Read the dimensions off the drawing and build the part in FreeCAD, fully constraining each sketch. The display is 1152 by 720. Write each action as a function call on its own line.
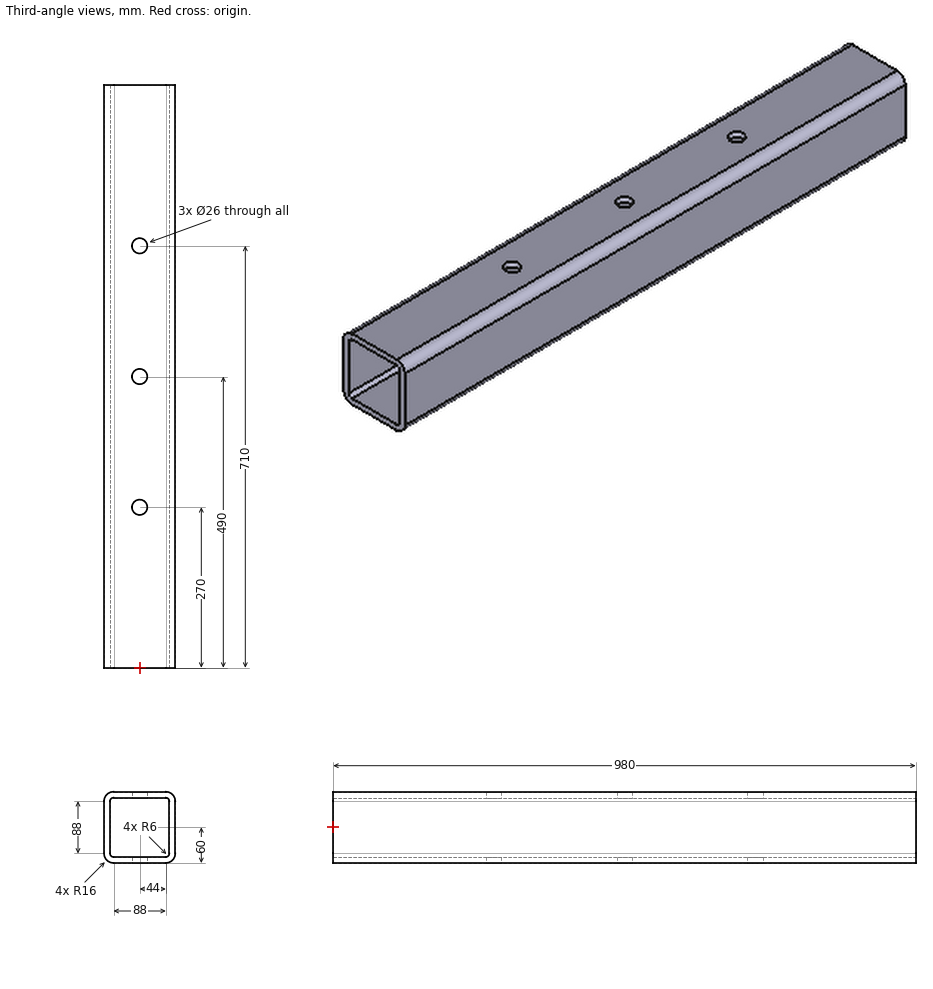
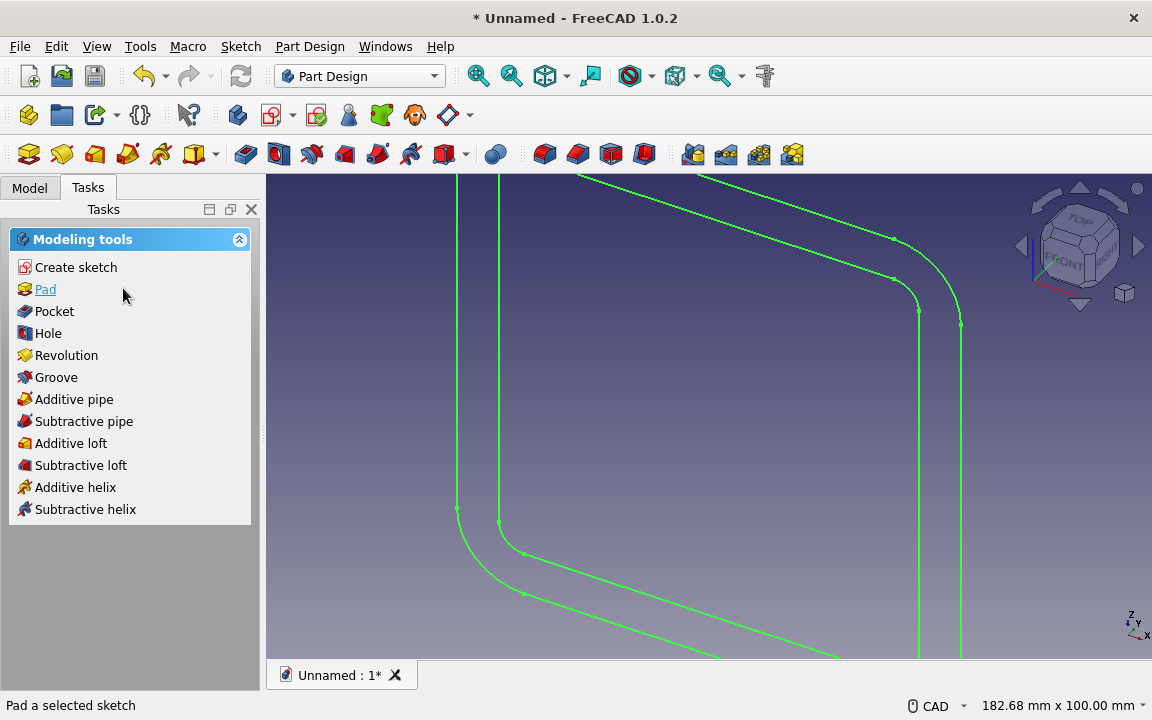
click(29, 154)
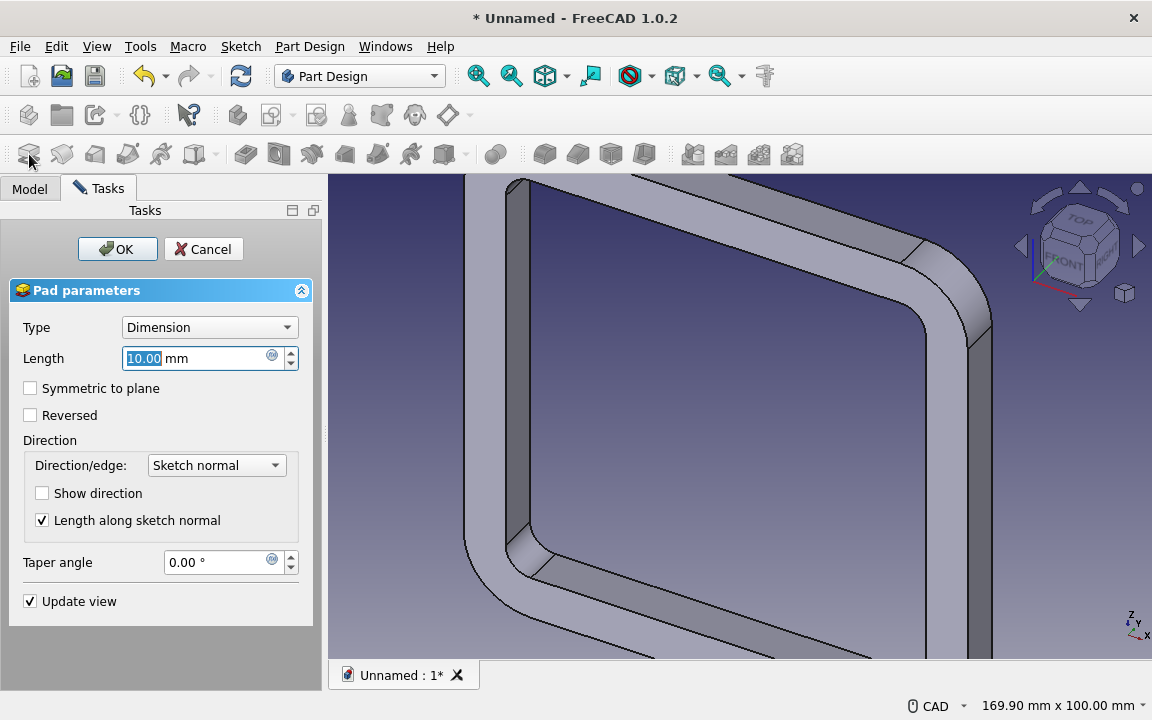
text(980)
key(Tab)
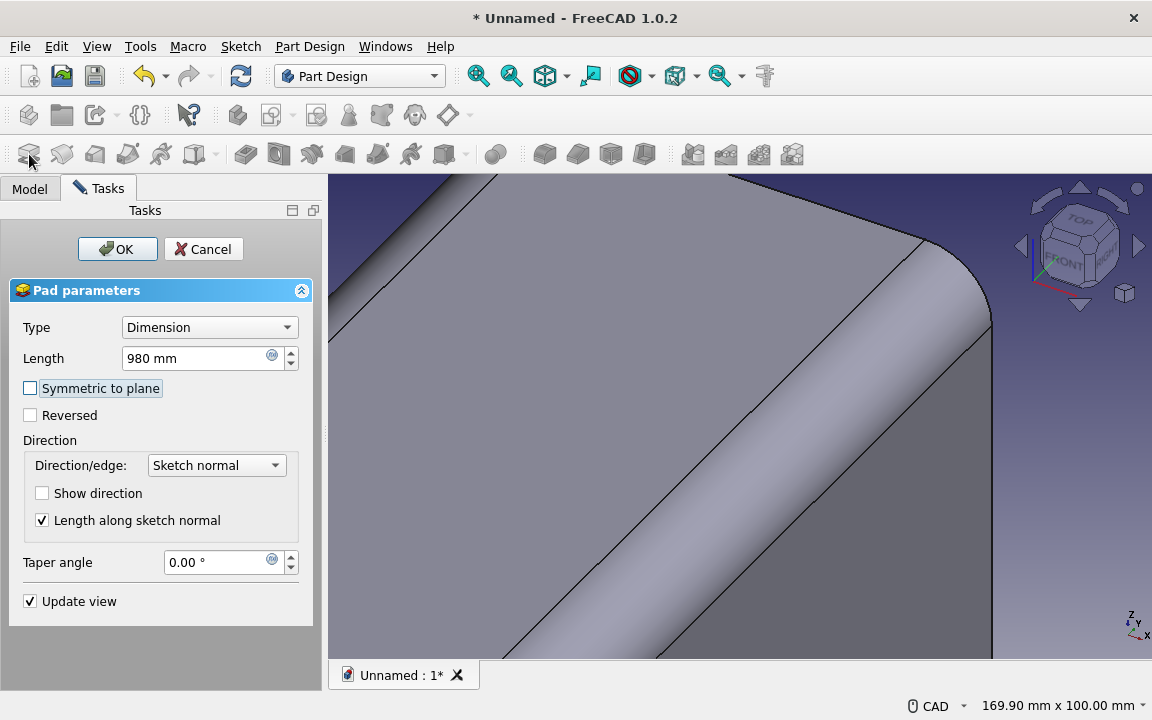
click(31, 415)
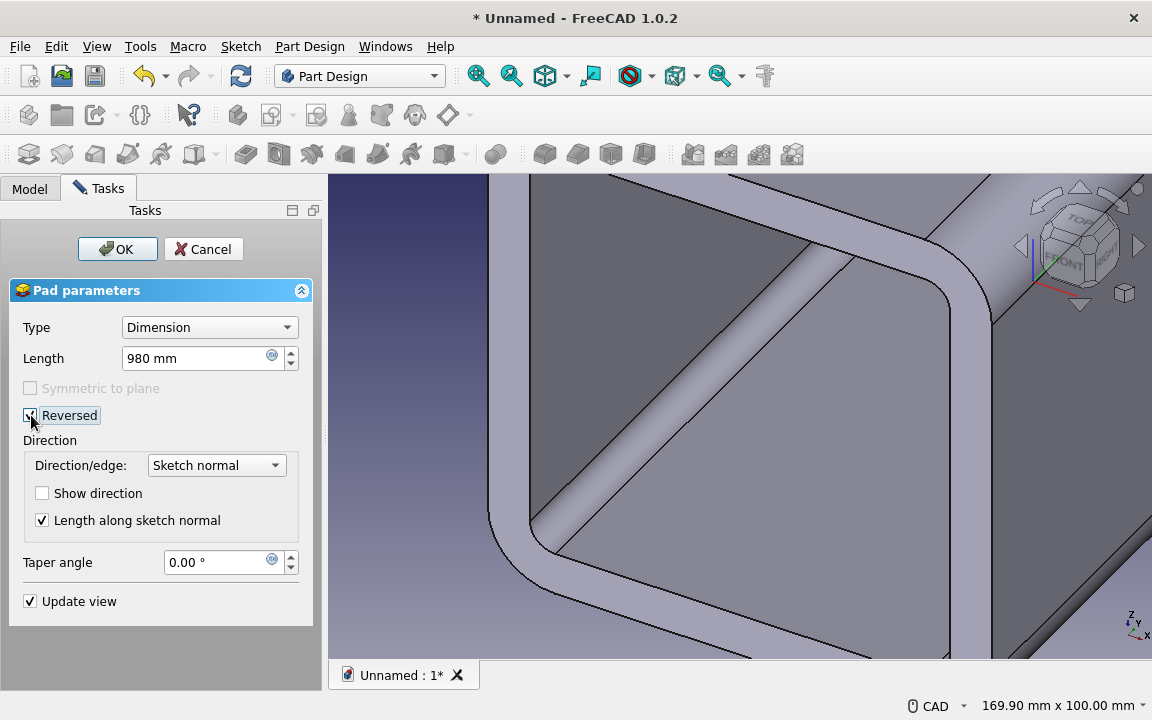
click(118, 249)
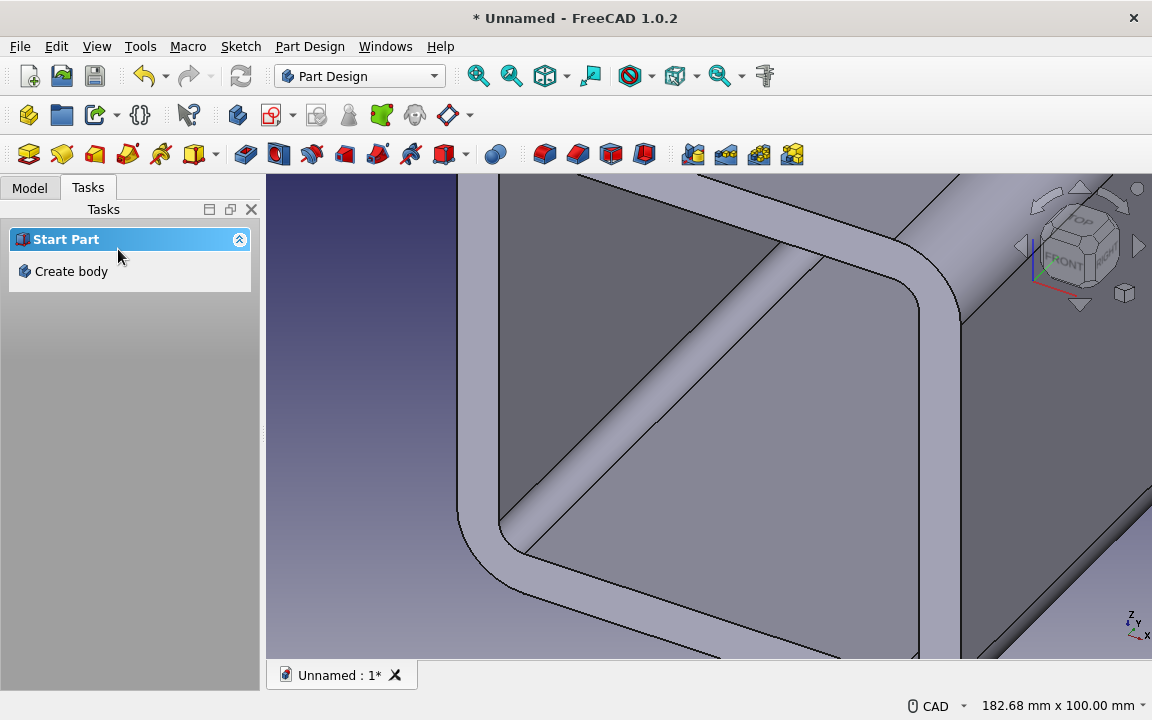
click(479, 76)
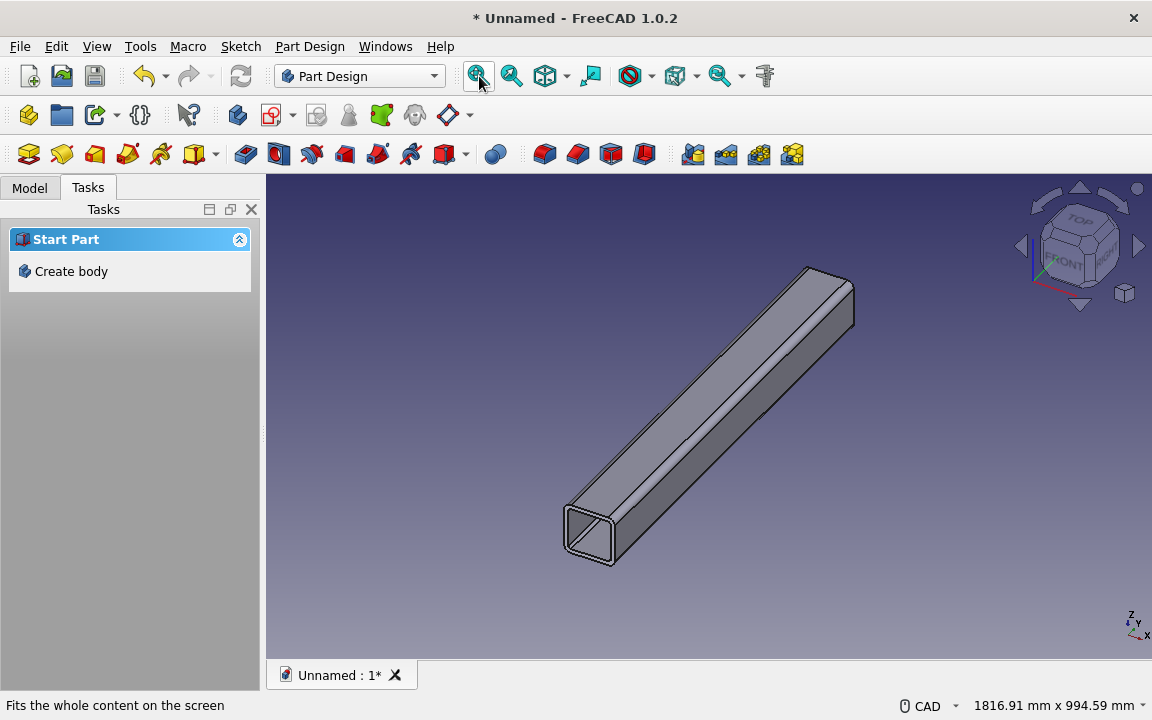
click(811, 290)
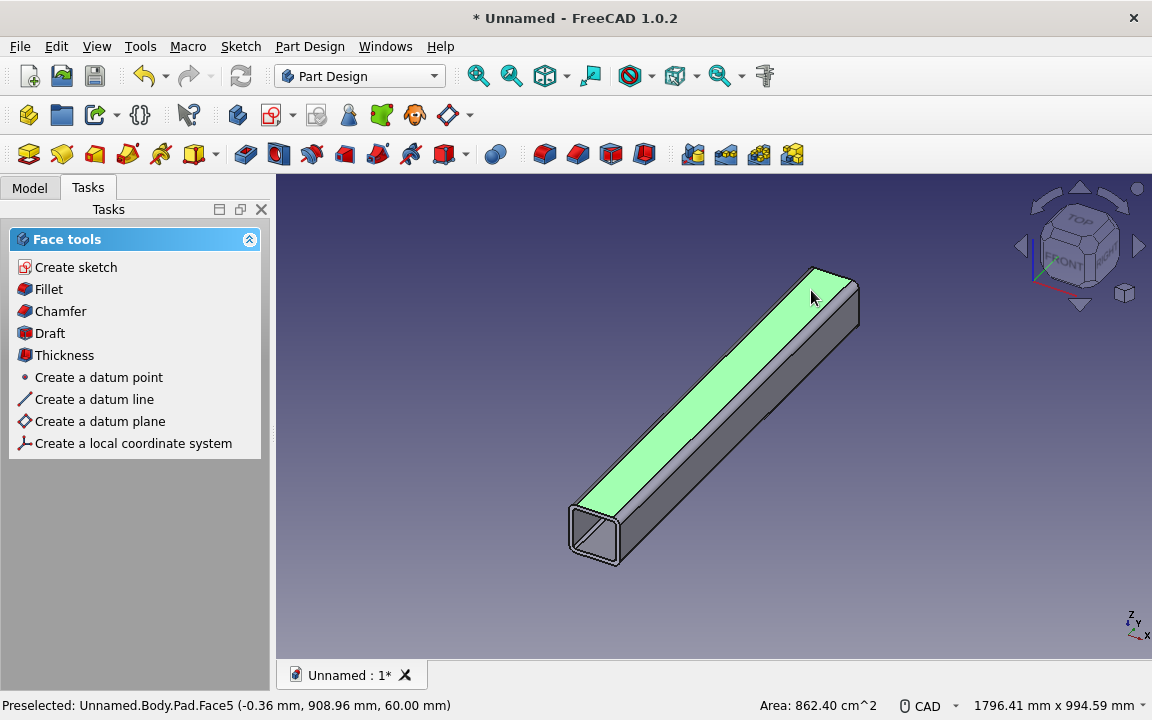
click(270, 116)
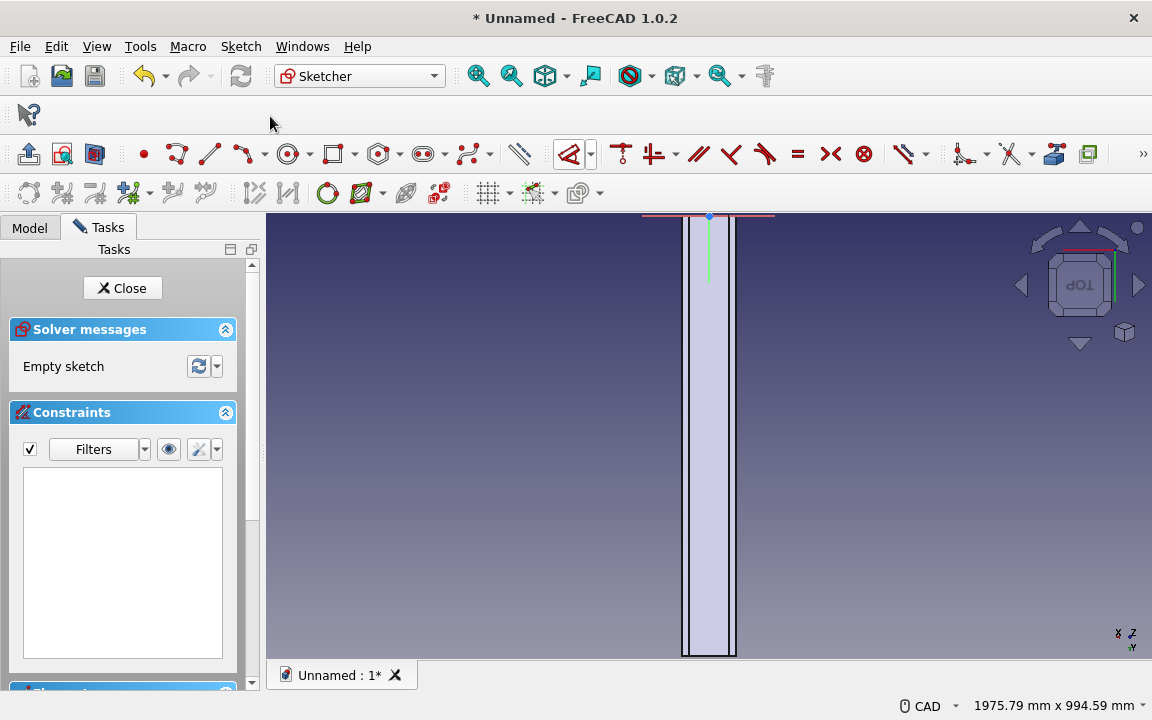
scroll(331, 631, down, 1)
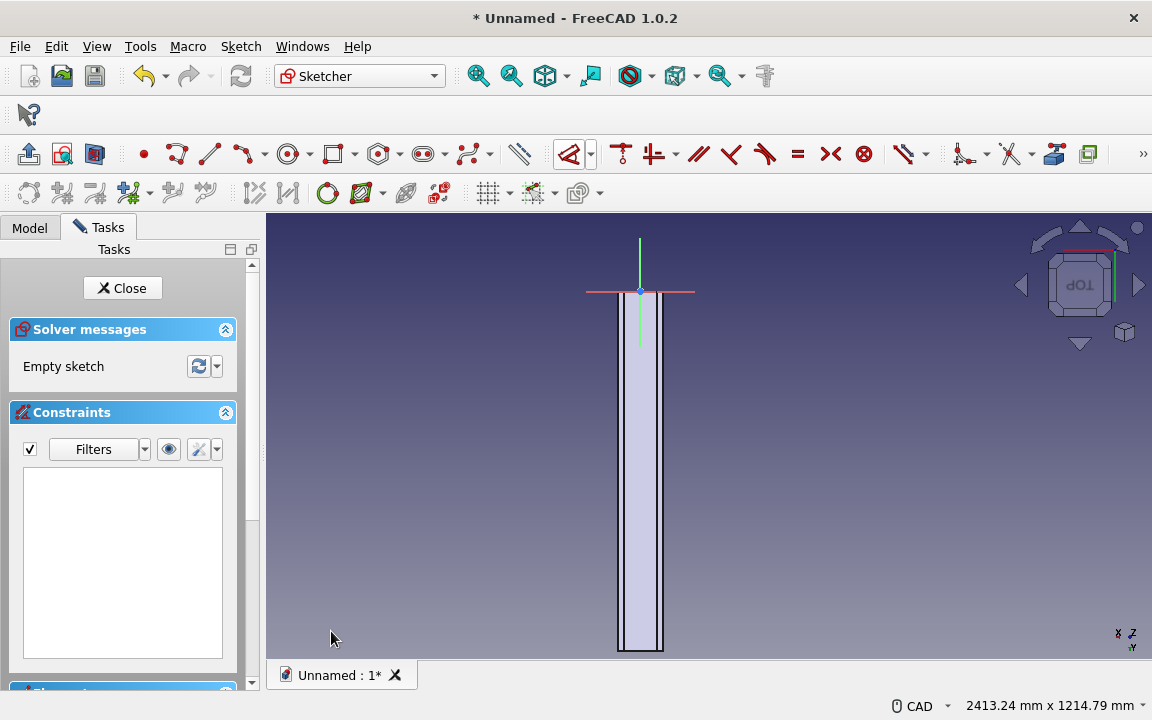
click(288, 154)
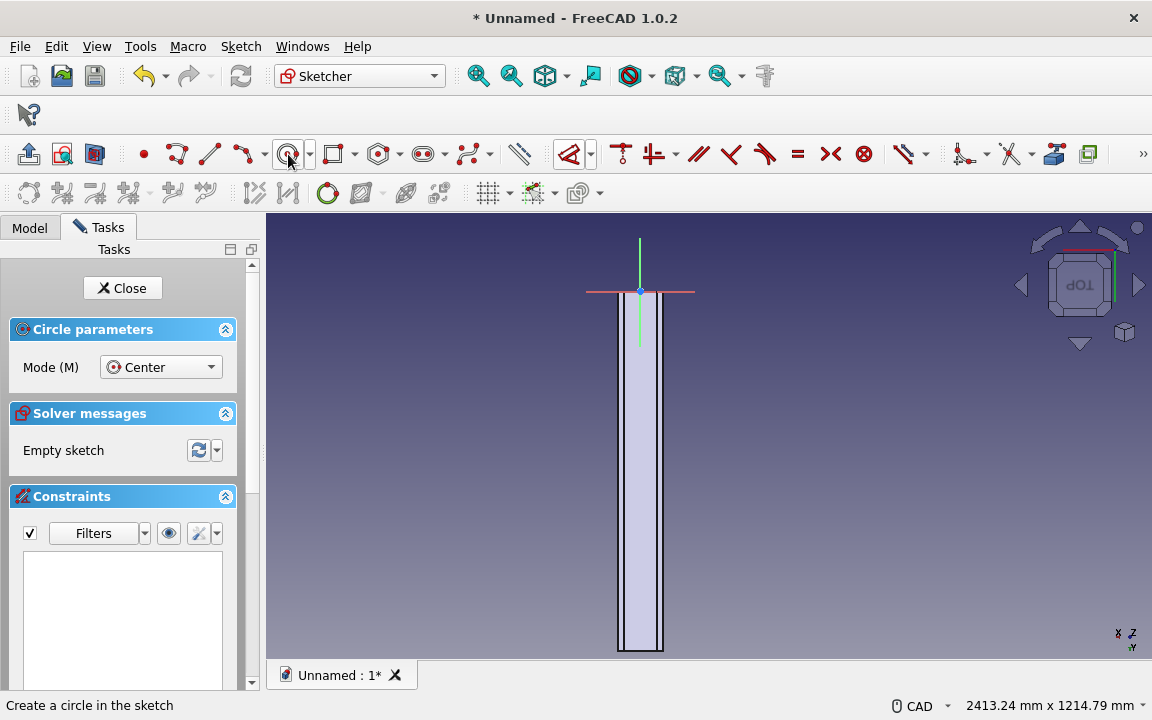
scroll(640, 552, up, 8)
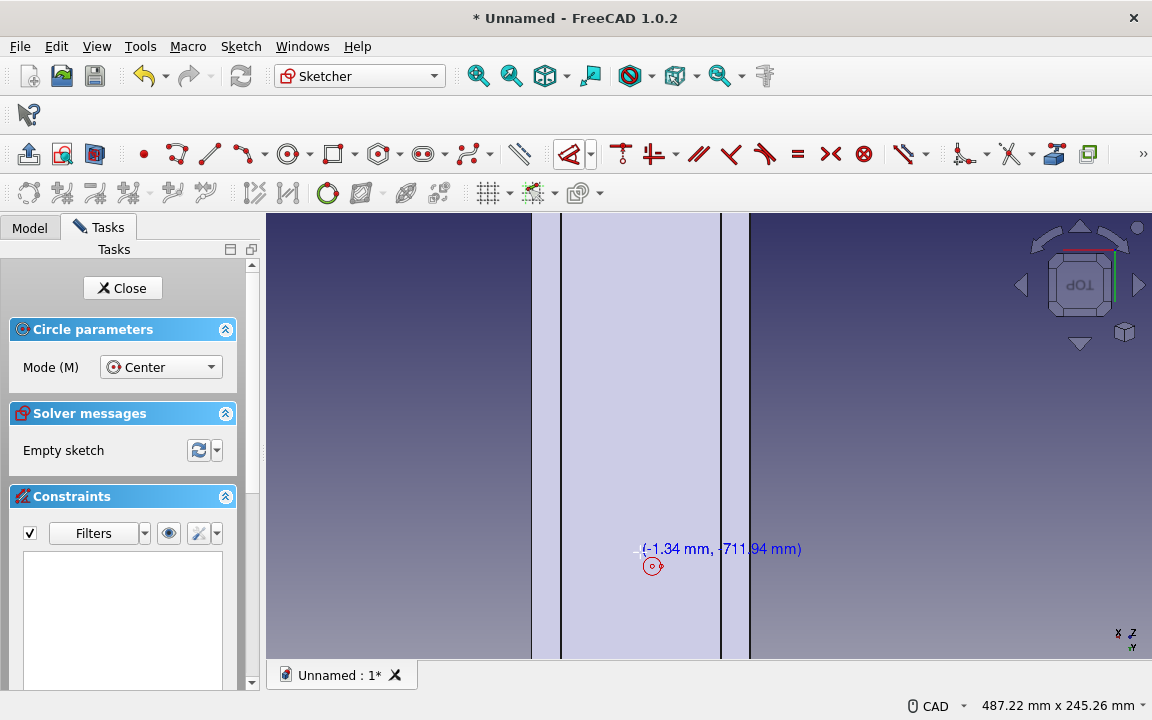
scroll(640, 567, down, 8)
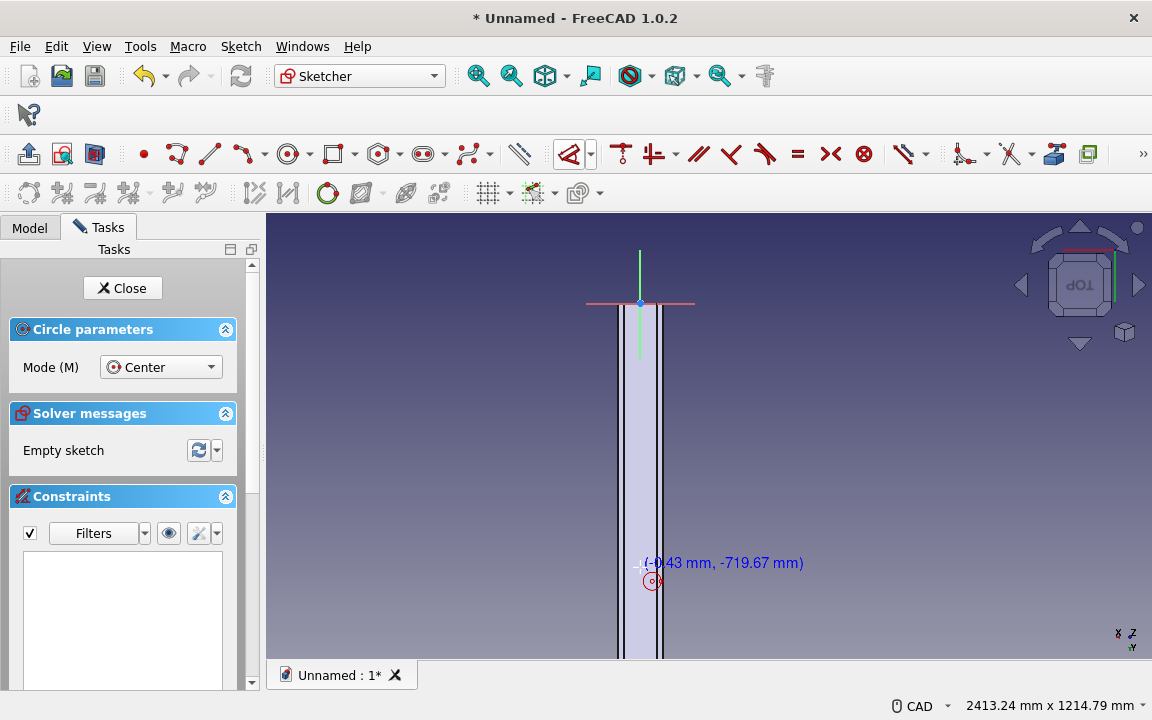
click(640, 564)